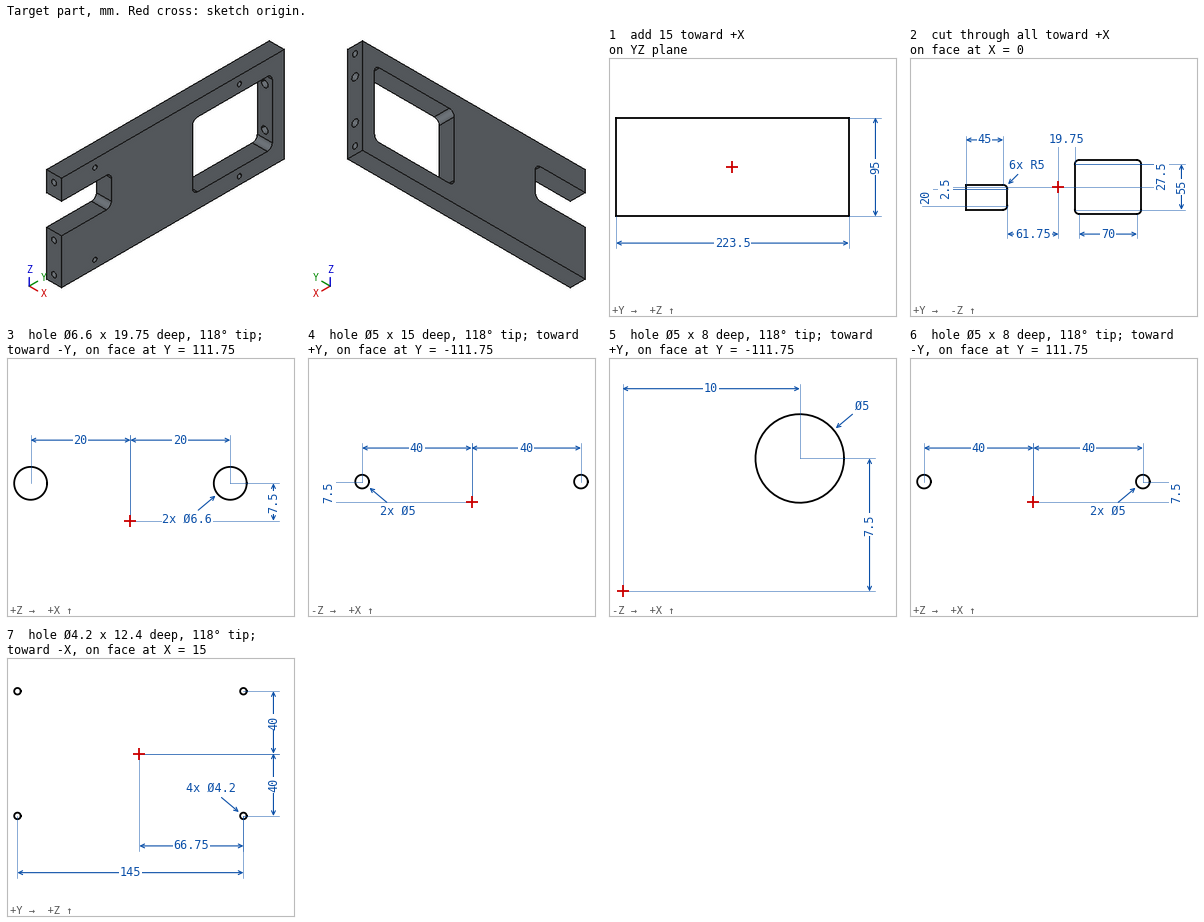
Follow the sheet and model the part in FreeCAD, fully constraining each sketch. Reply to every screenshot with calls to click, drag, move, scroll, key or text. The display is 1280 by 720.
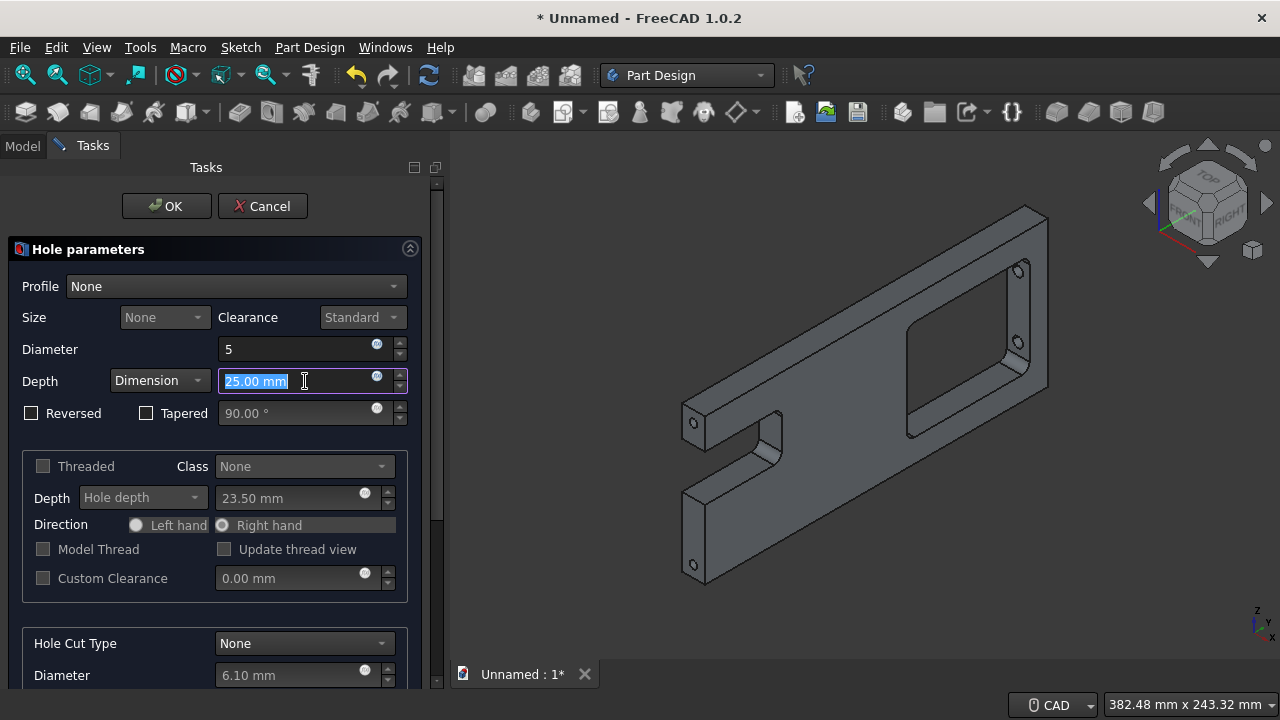
text(15)
key(Tab)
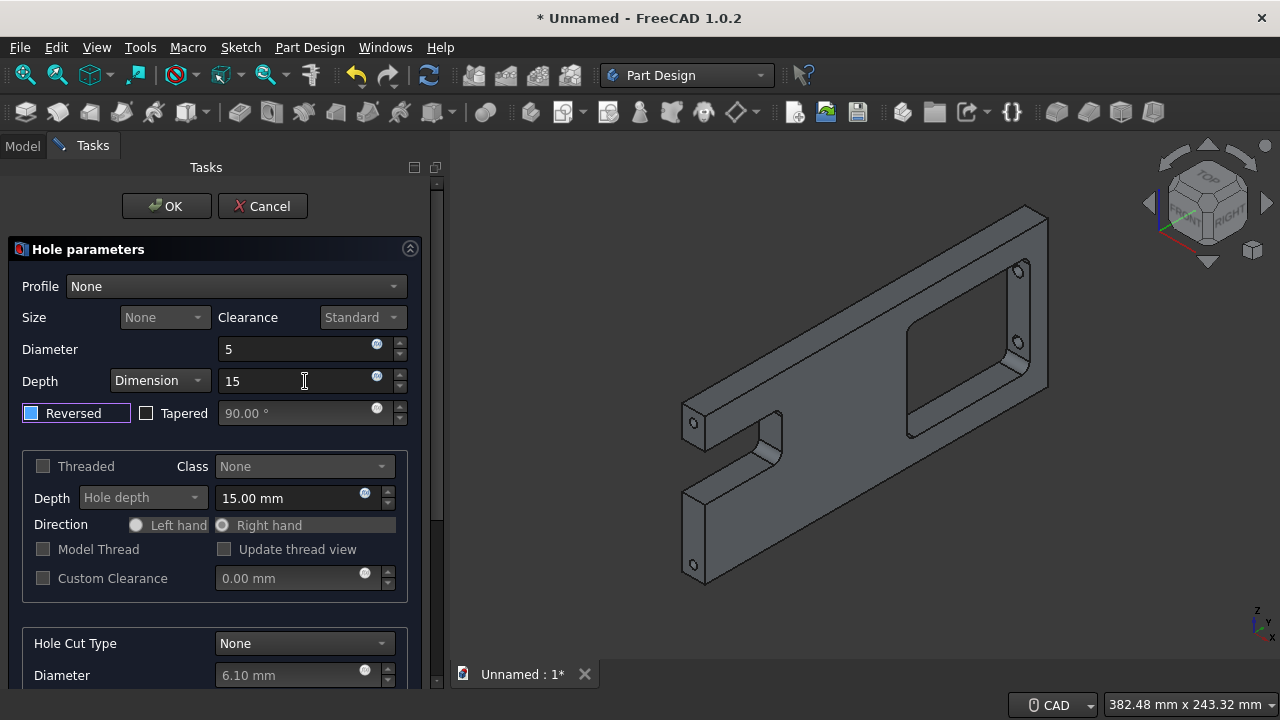
click(167, 206)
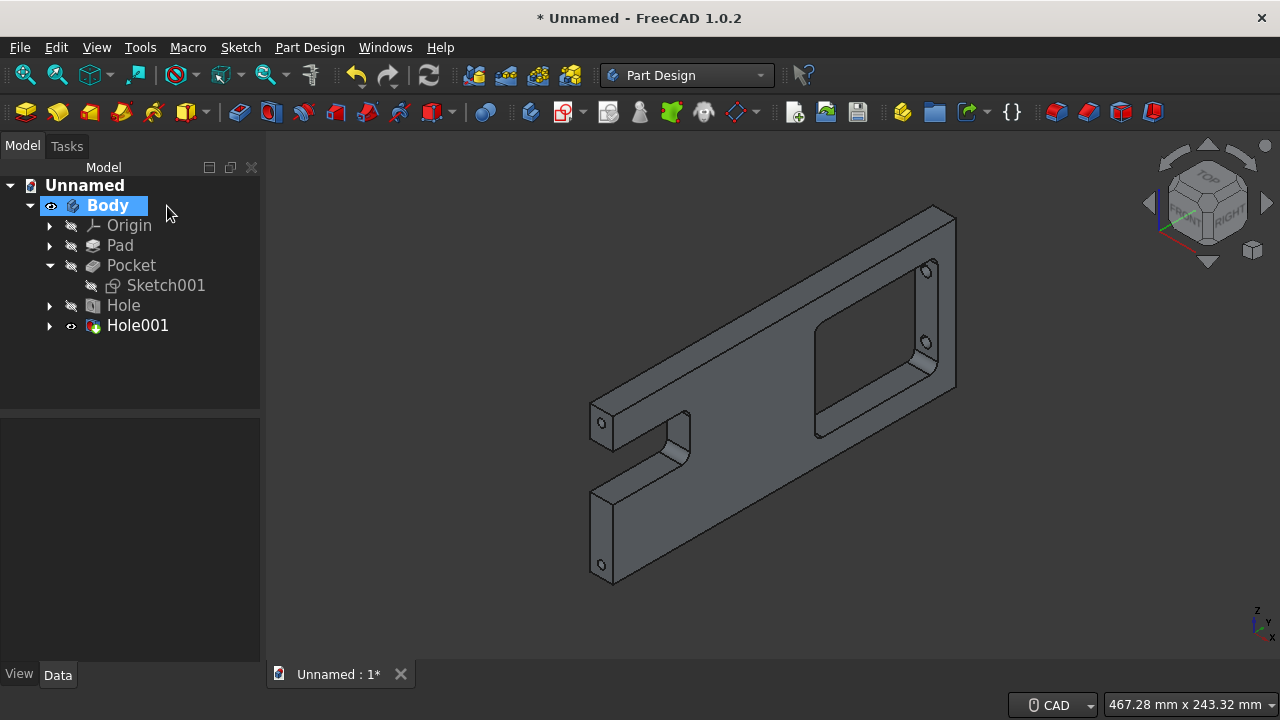
click(602, 526)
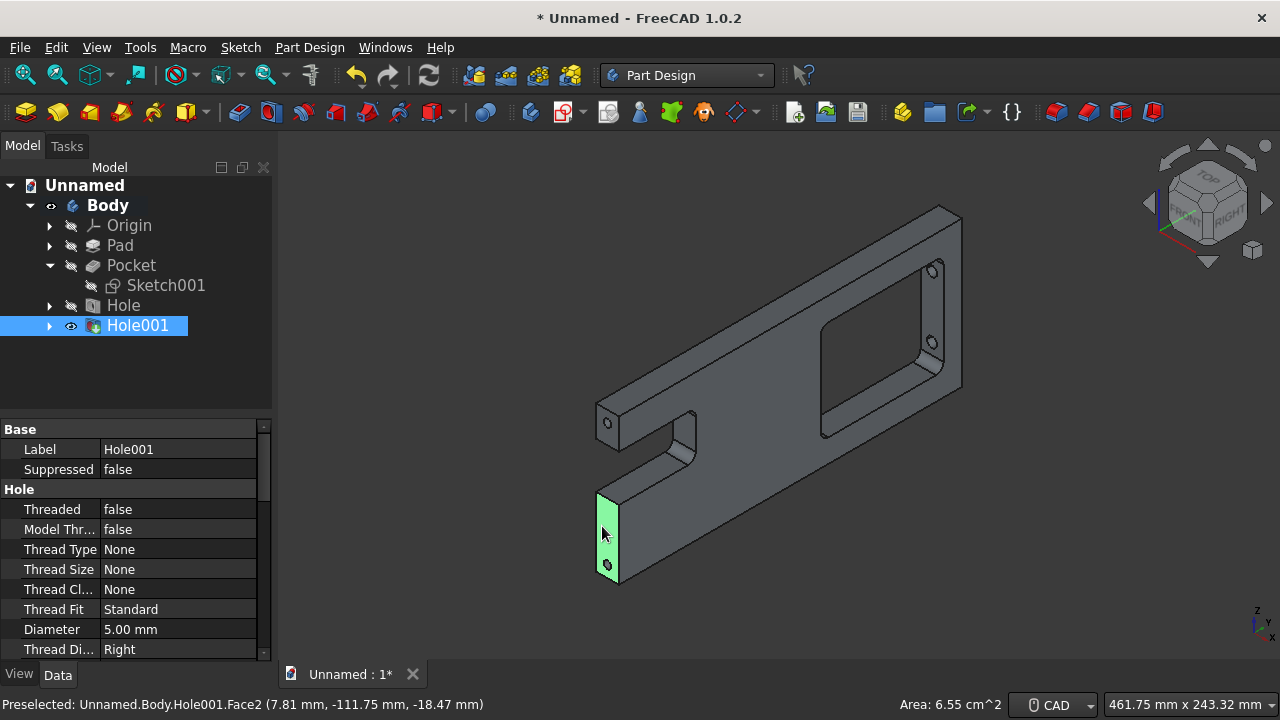
click(564, 112)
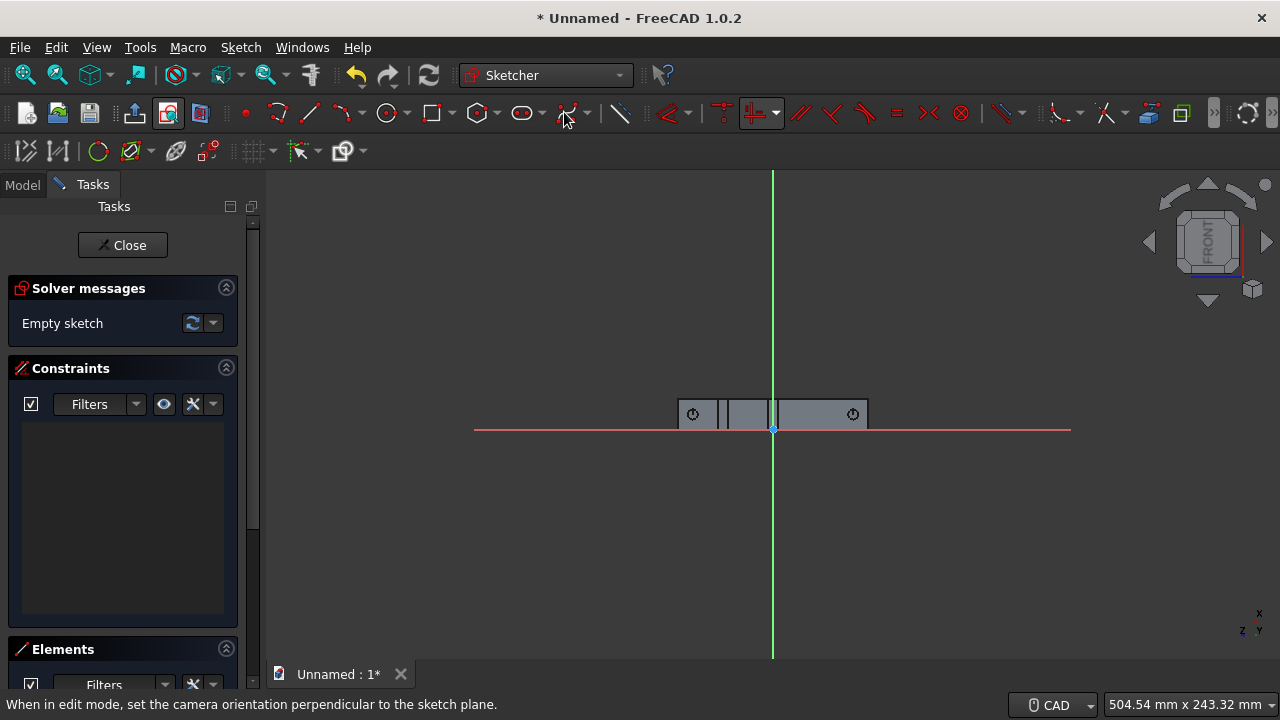
scroll(798, 414, up, 15)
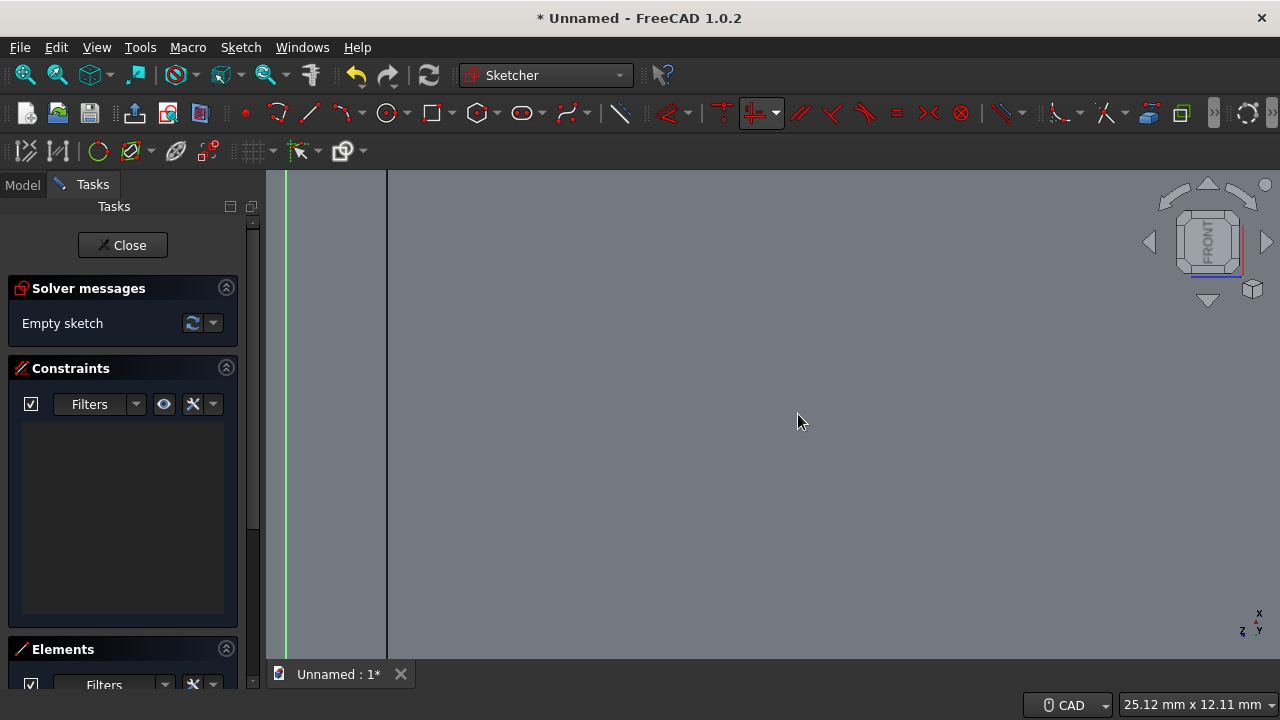
scroll(659, 415, up, 2)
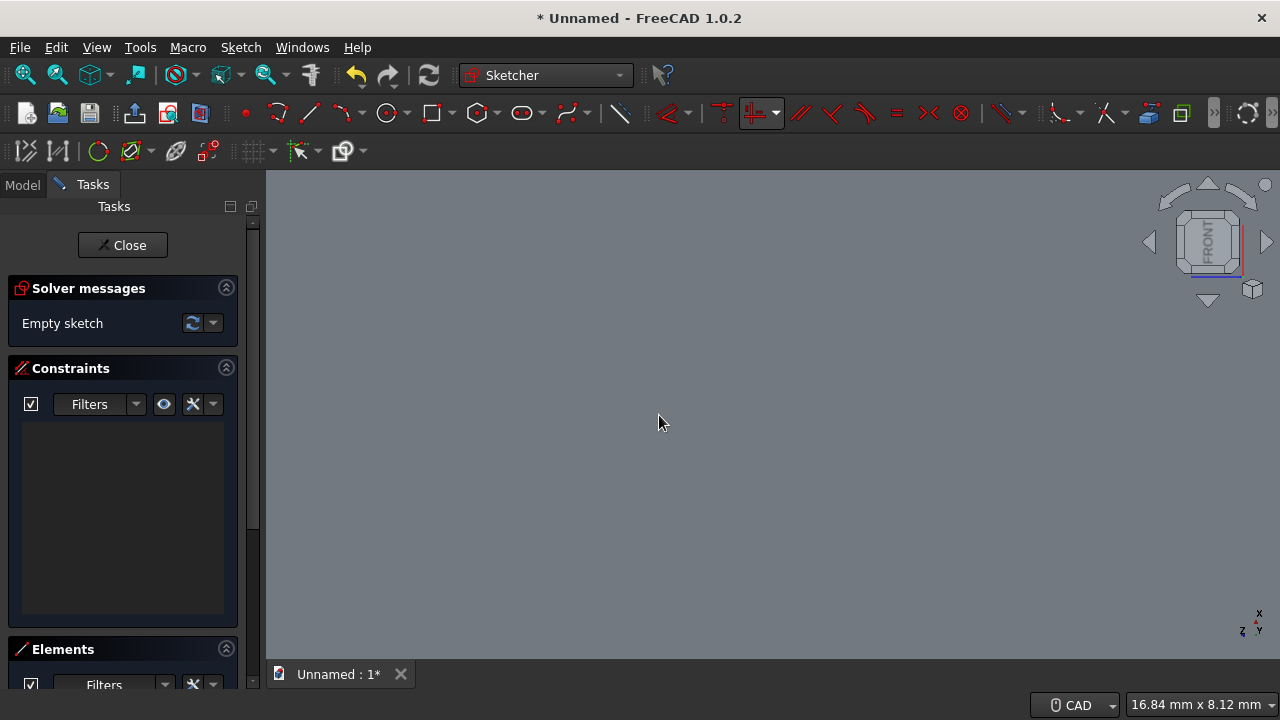
click(388, 114)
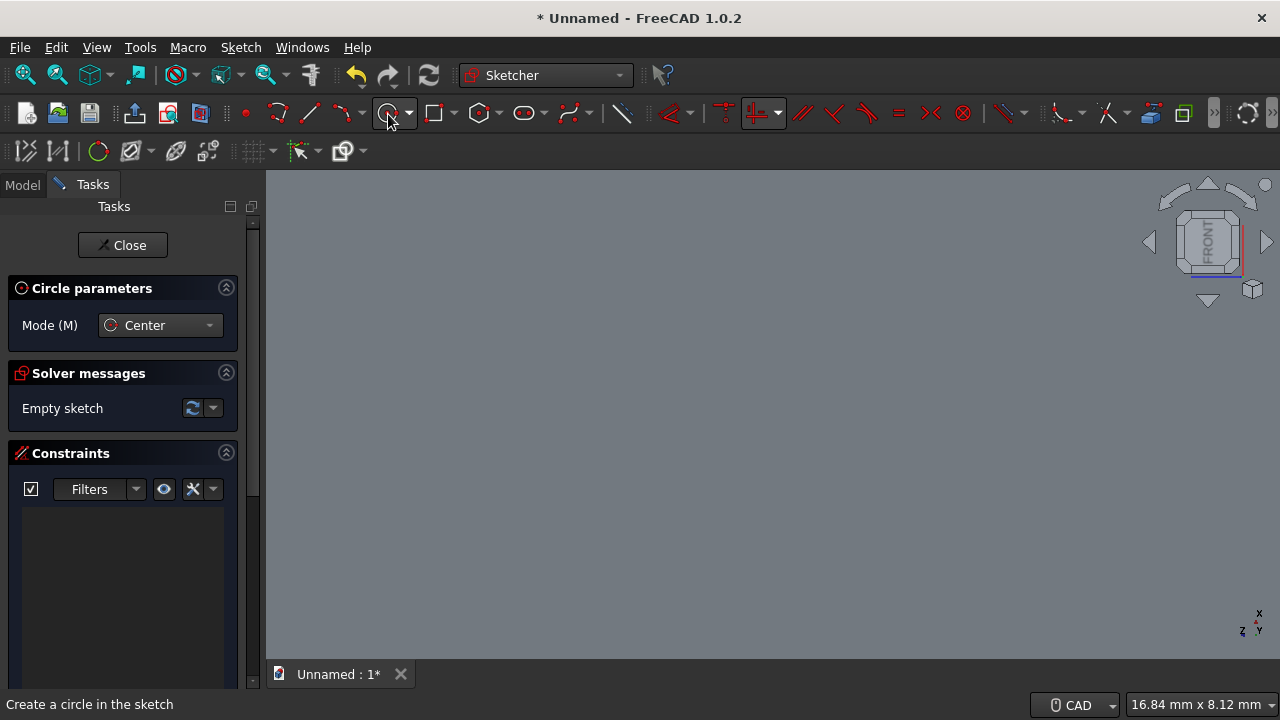
click(704, 414)
move(811, 308)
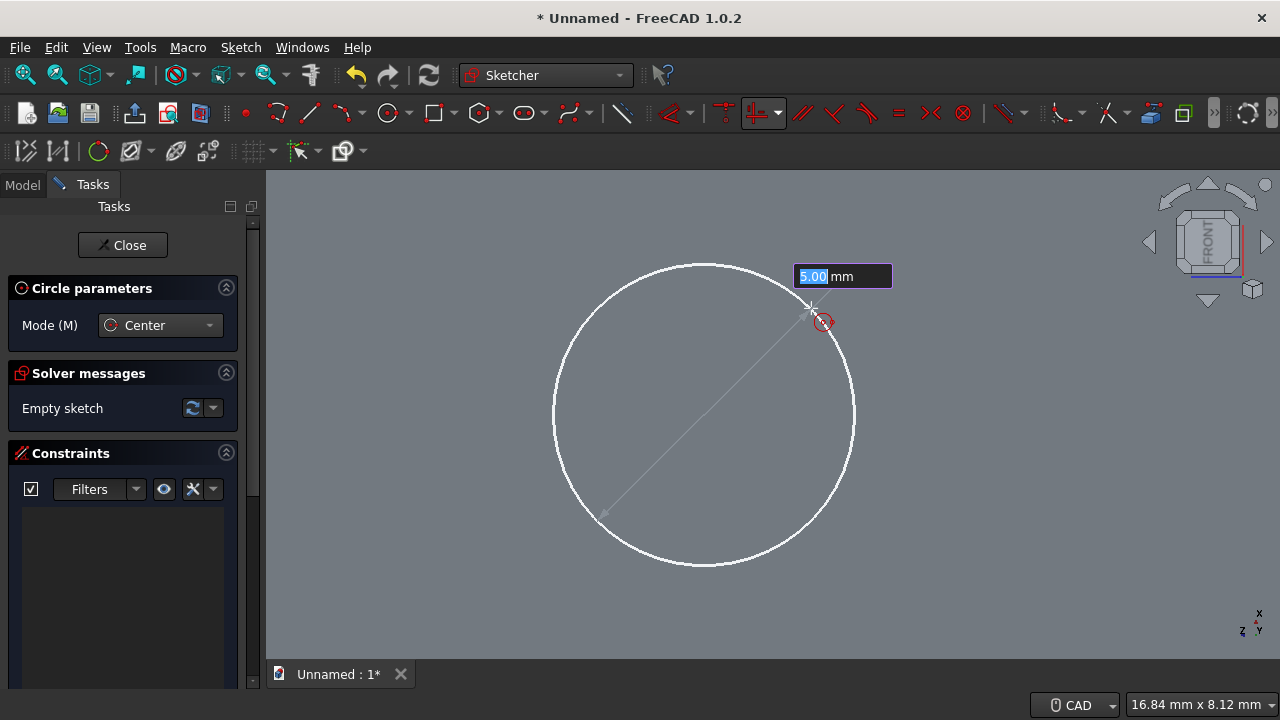
text(5)
key(Return)
key(Escape)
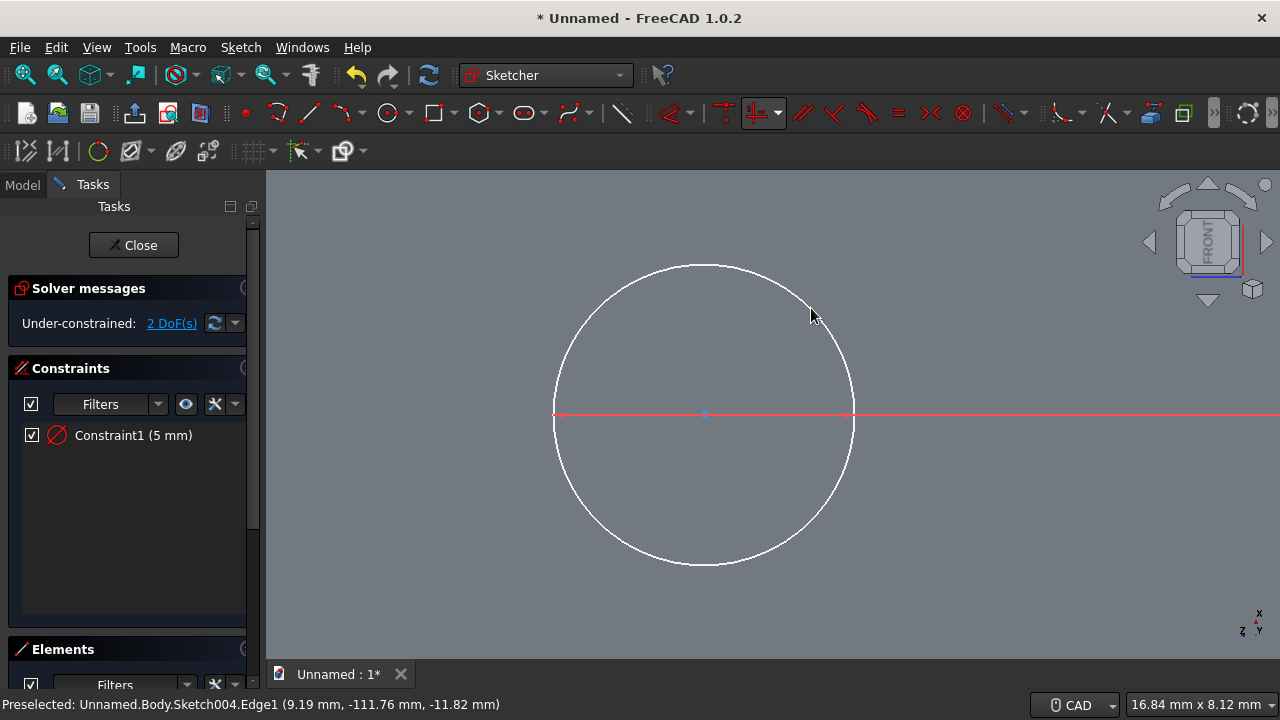
click(670, 114)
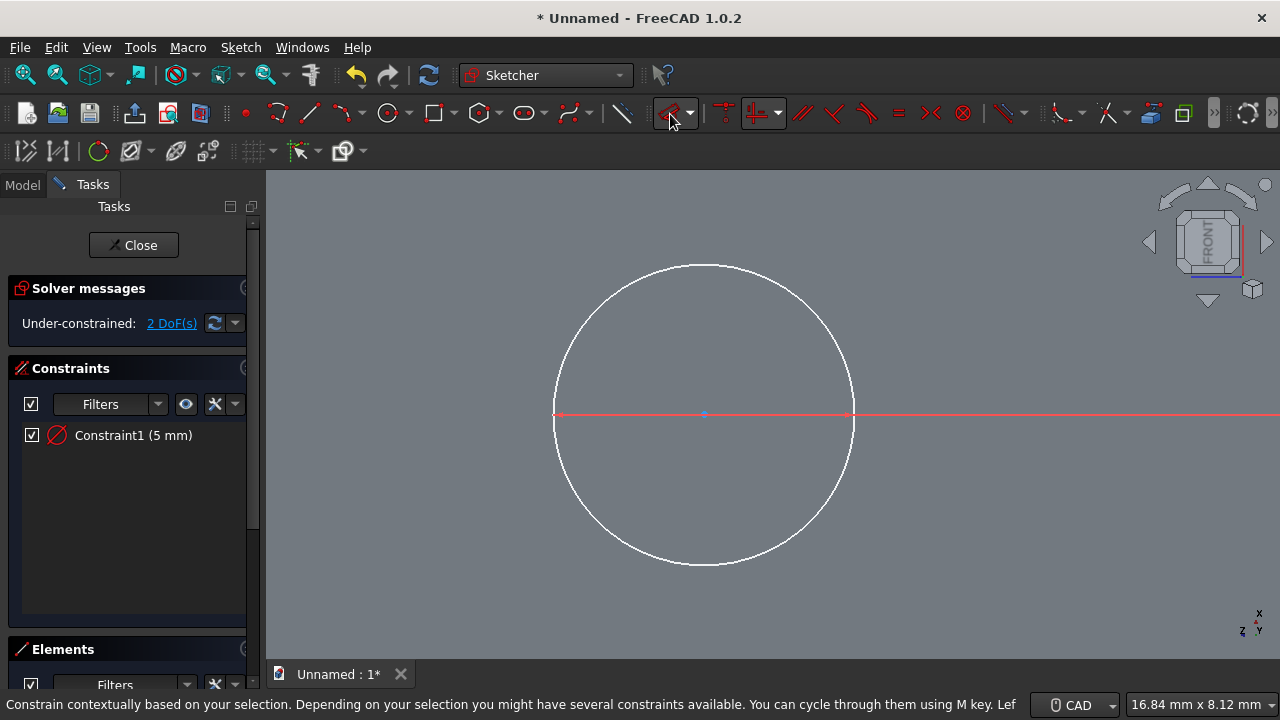
click(704, 415)
click(499, 381)